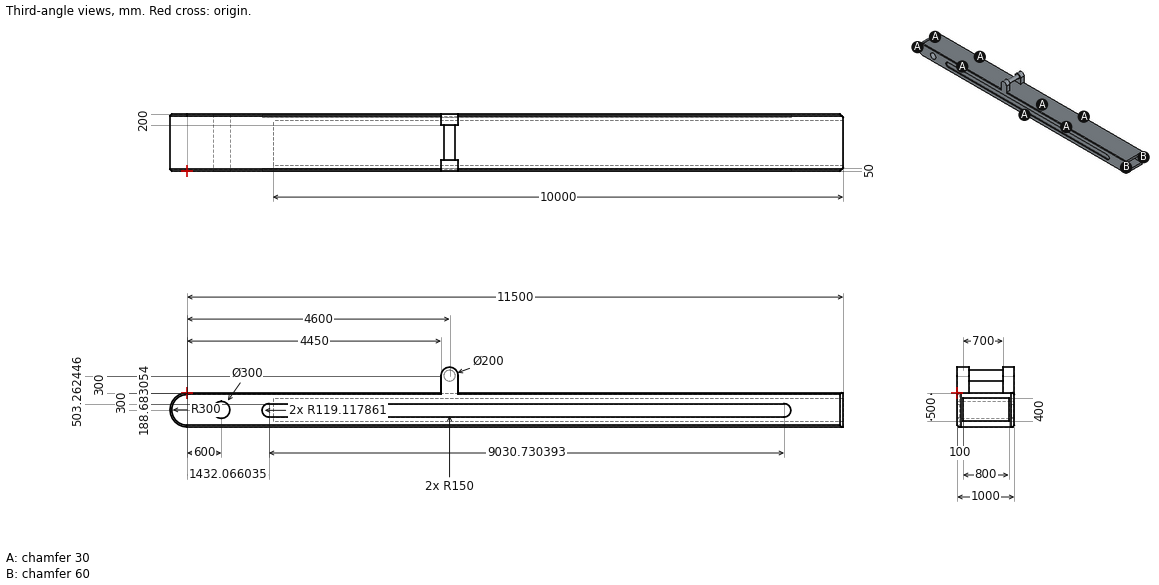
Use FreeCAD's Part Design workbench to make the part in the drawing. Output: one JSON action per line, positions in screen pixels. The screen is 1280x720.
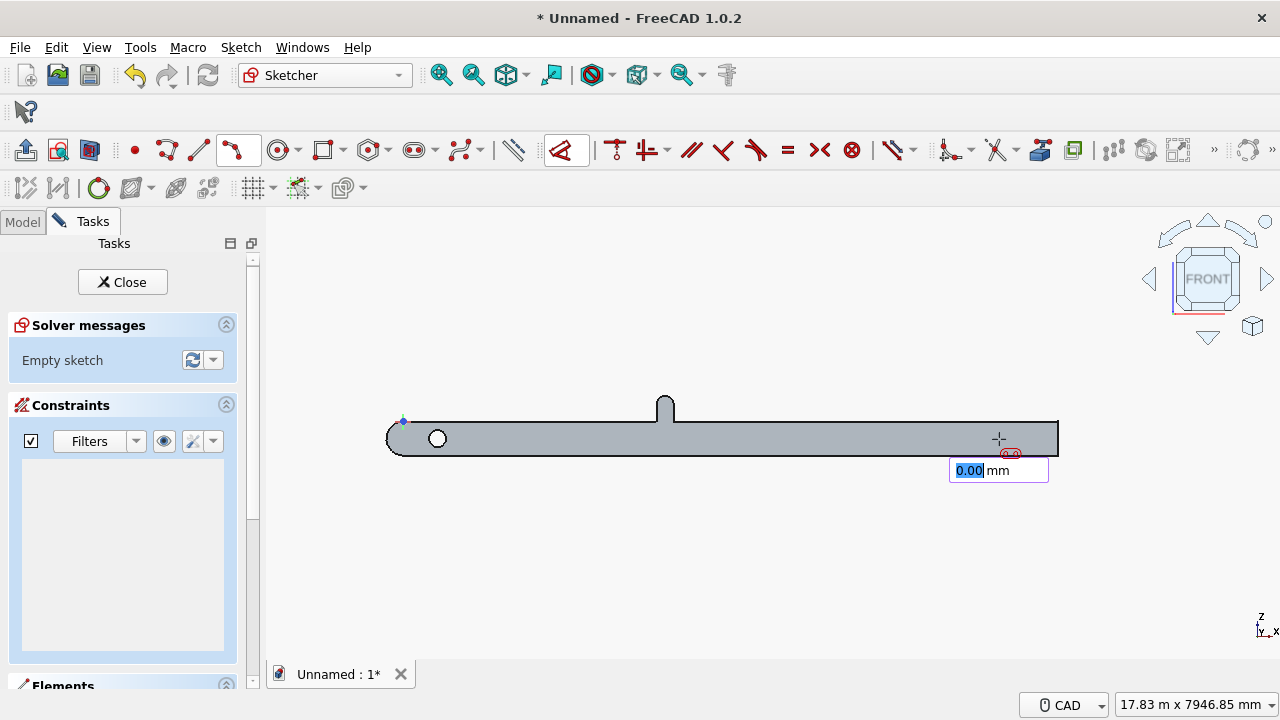
{"action": "scroll", "coordinate": [742, 446], "scroll_direction": "up", "scroll_amount": 5}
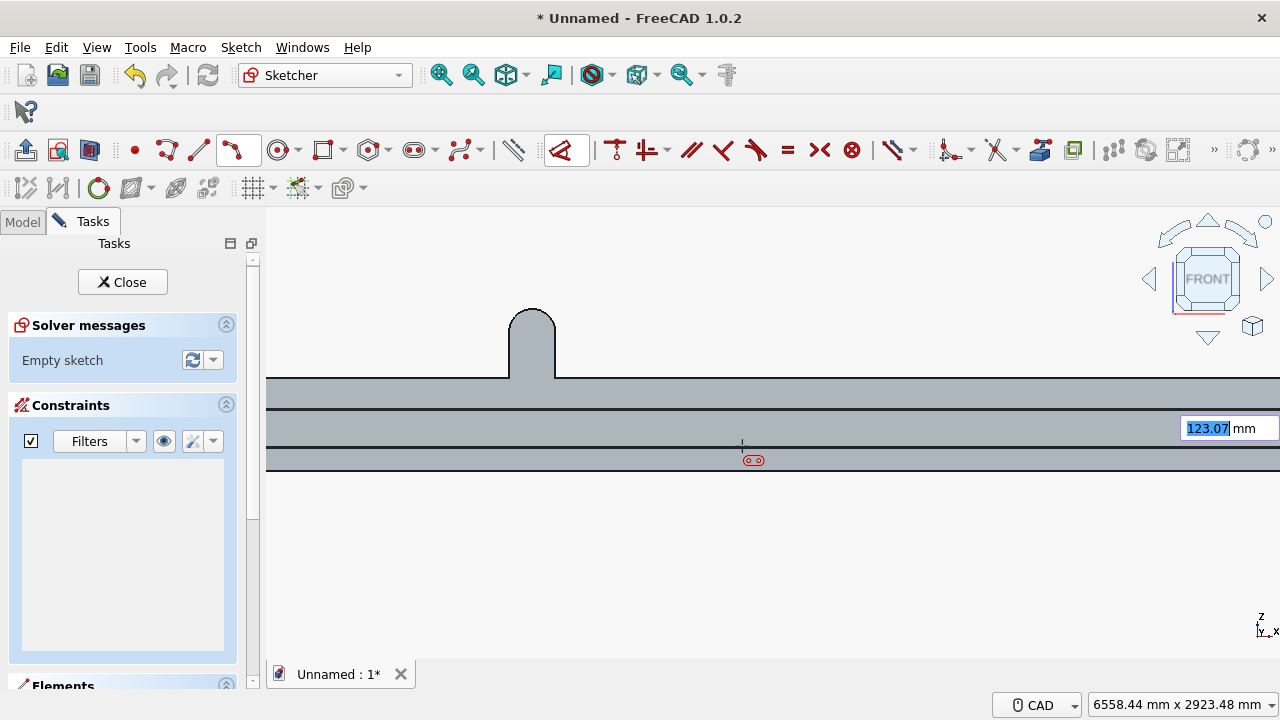
{"action": "left_click", "coordinate": [740, 444]}
{"action": "key", "text": "Escape"}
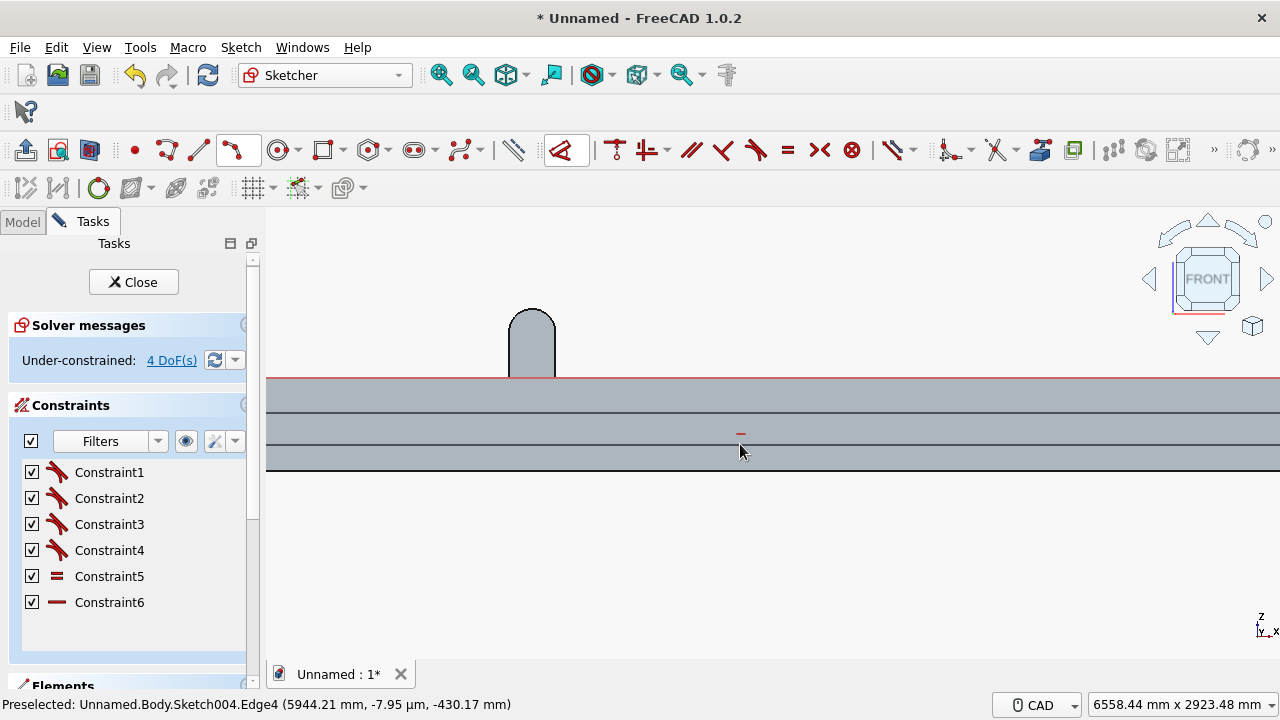
{"action": "scroll", "coordinate": [743, 446], "scroll_direction": "down", "scroll_amount": 5}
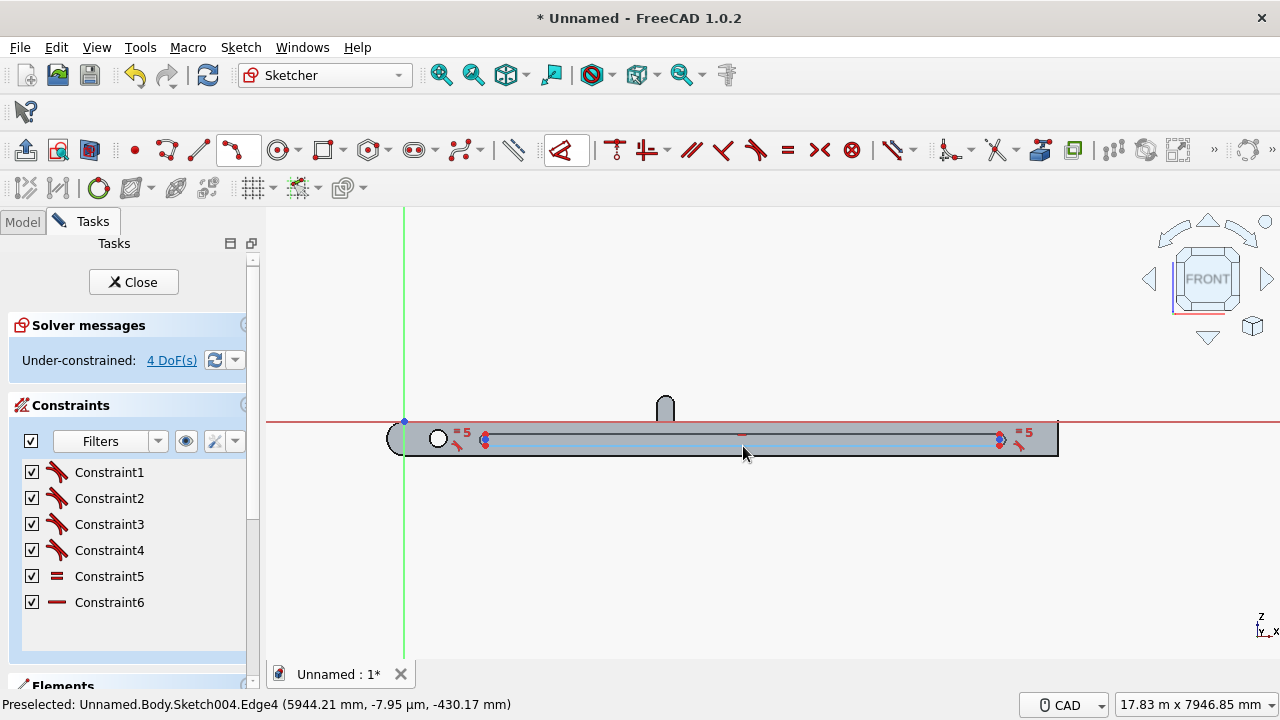
{"action": "scroll", "coordinate": [481, 436], "scroll_direction": "up", "scroll_amount": 9}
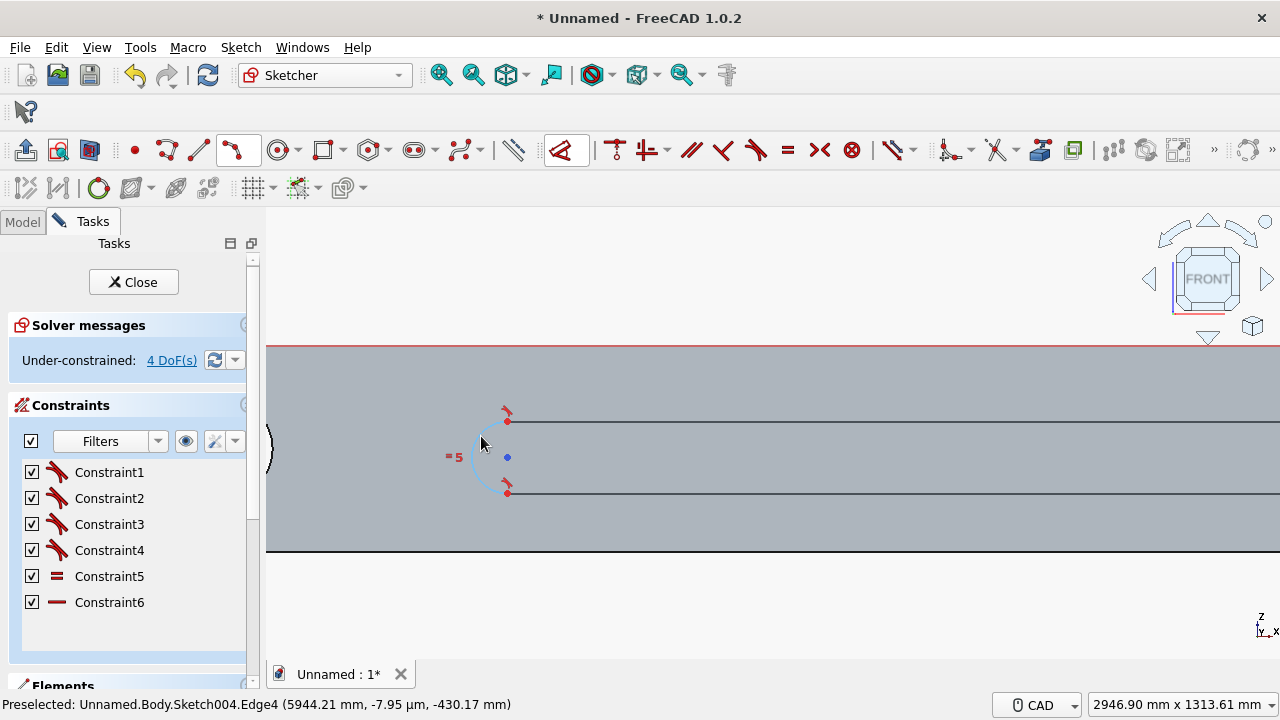
{"action": "left_click", "coordinate": [479, 436]}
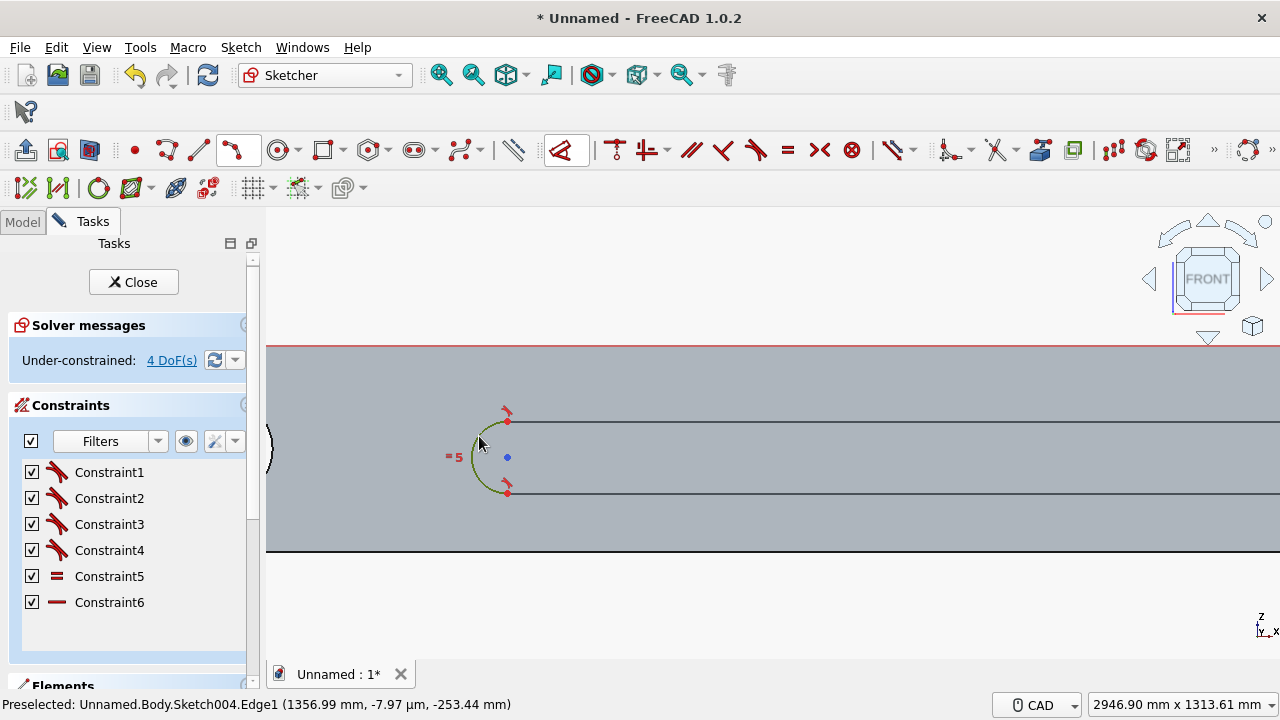
{"action": "left_click", "coordinate": [584, 150]}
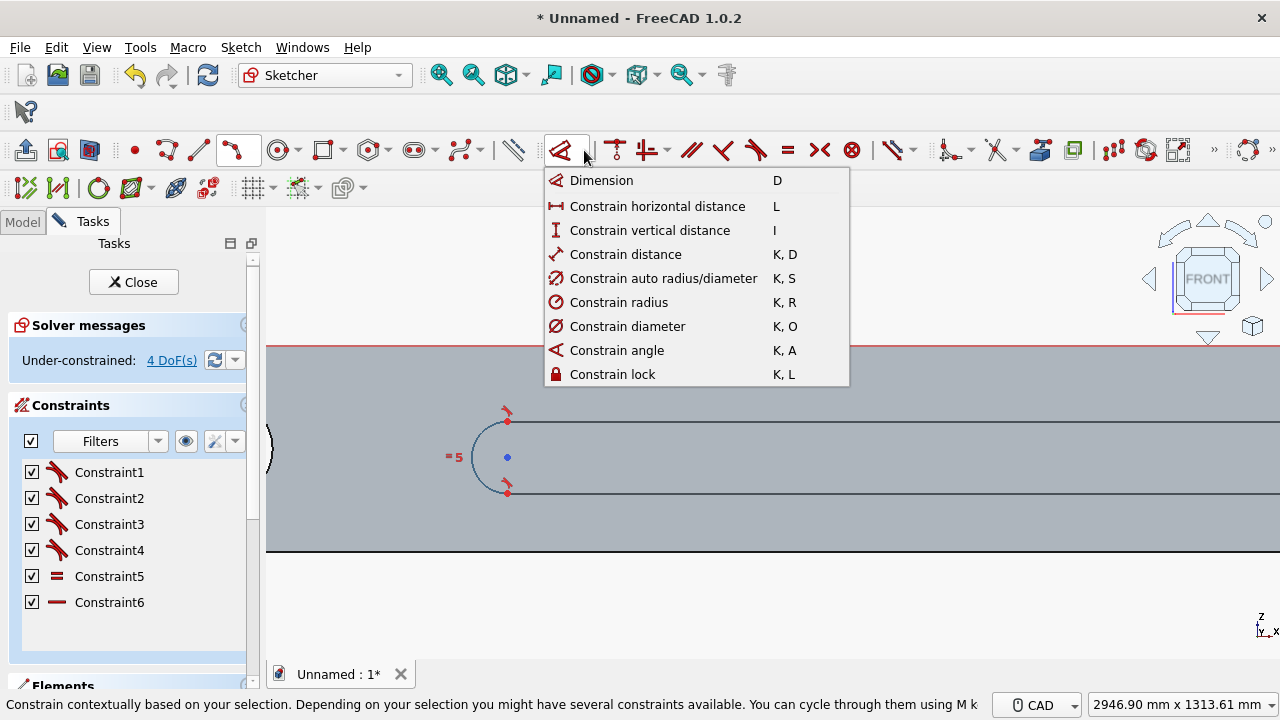
{"action": "left_click", "coordinate": [697, 302]}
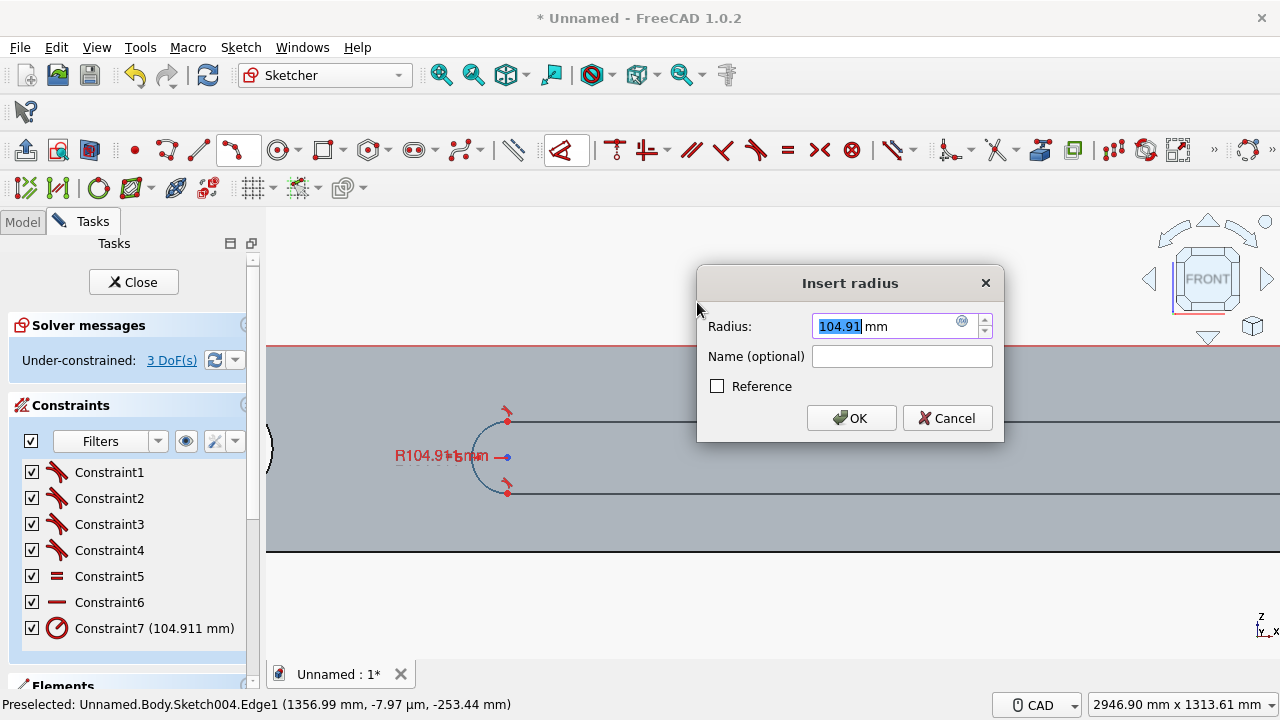
{"action": "type", "text": "119.117861"}
{"action": "key", "text": "Return"}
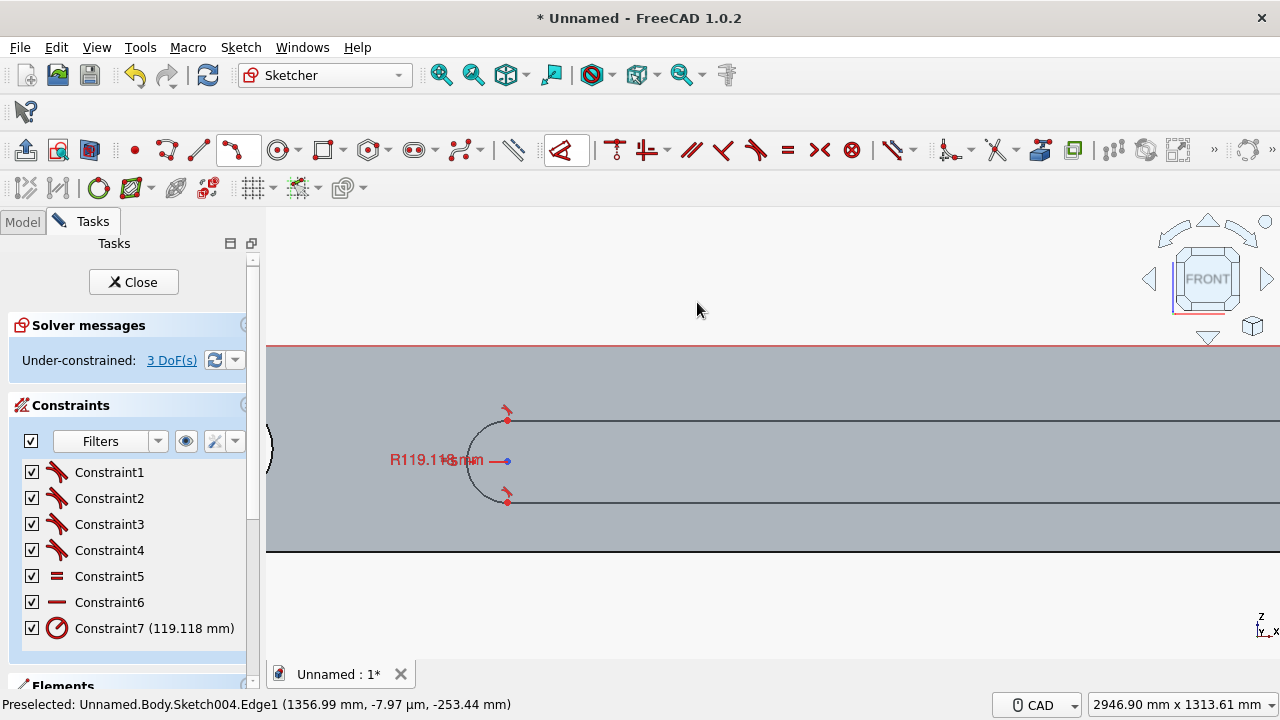
{"action": "scroll", "coordinate": [481, 436], "scroll_direction": "down", "scroll_amount": 9}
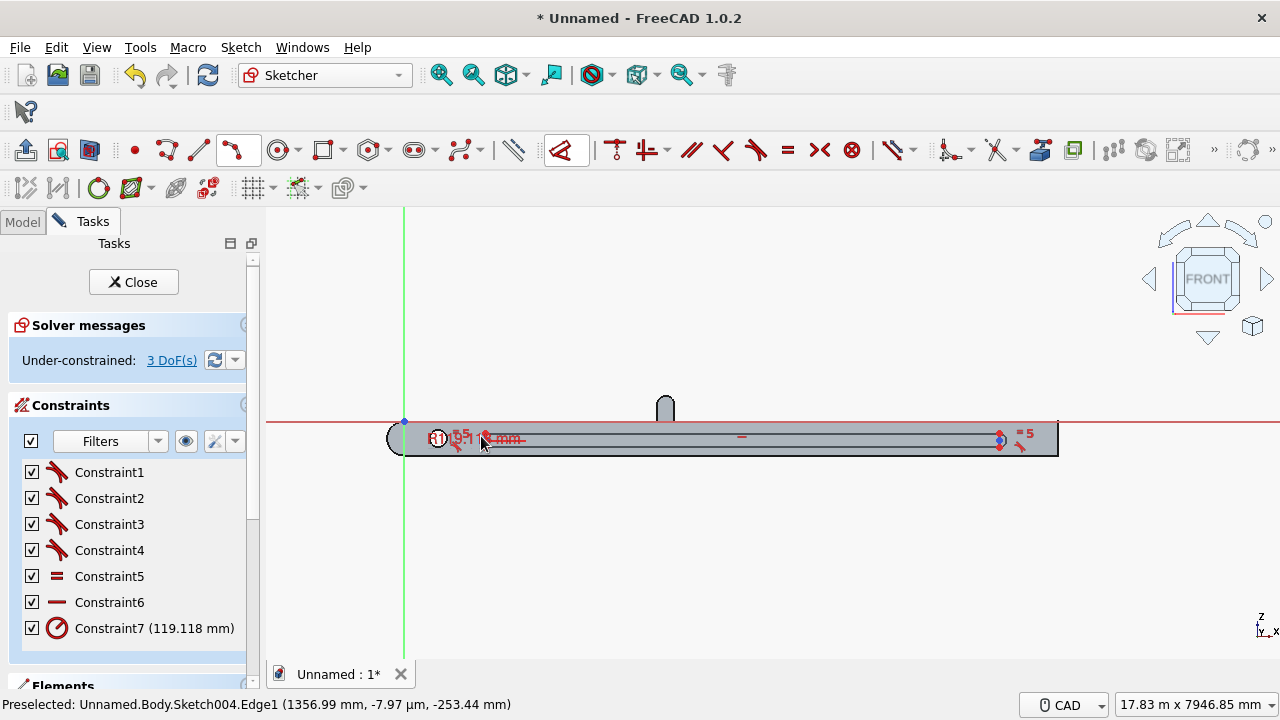
{"action": "left_click", "coordinate": [640, 434]}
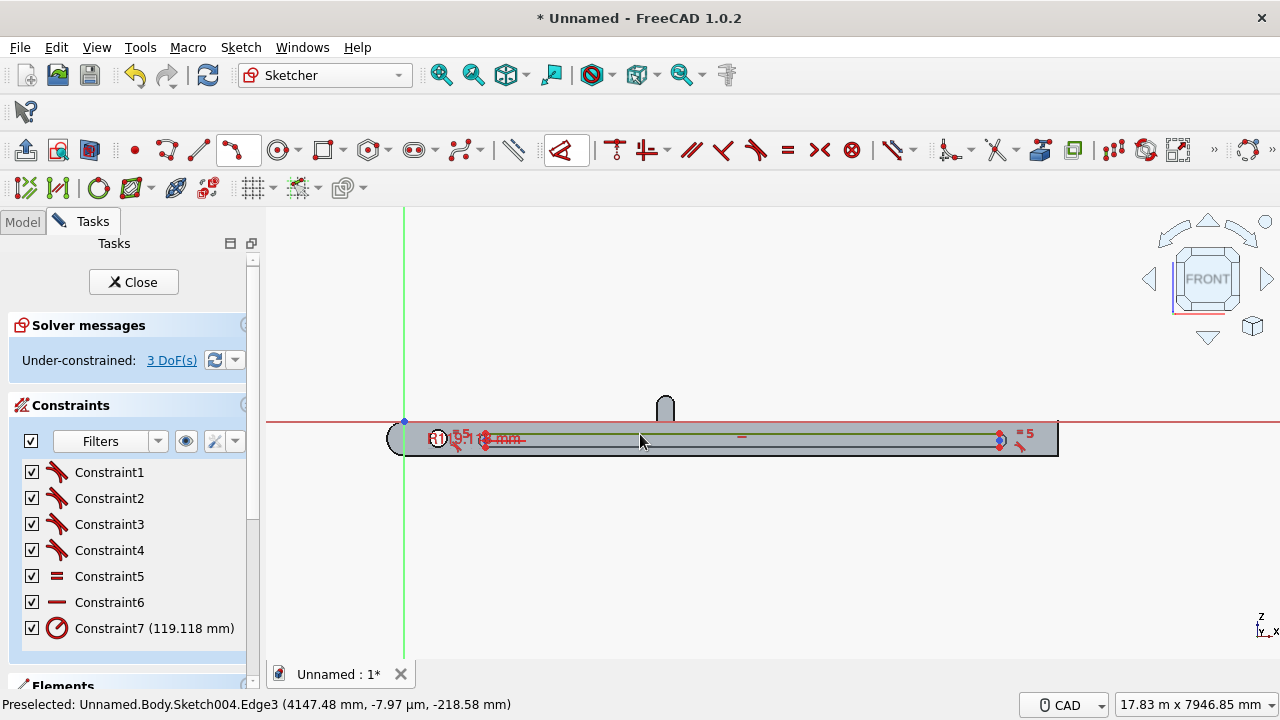
{"action": "left_click", "coordinate": [584, 150]}